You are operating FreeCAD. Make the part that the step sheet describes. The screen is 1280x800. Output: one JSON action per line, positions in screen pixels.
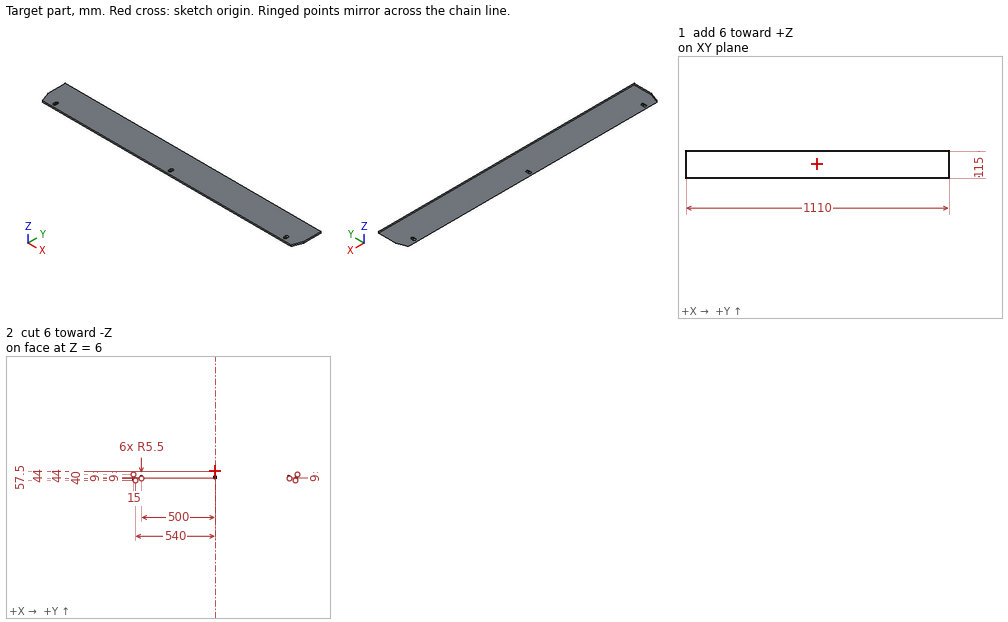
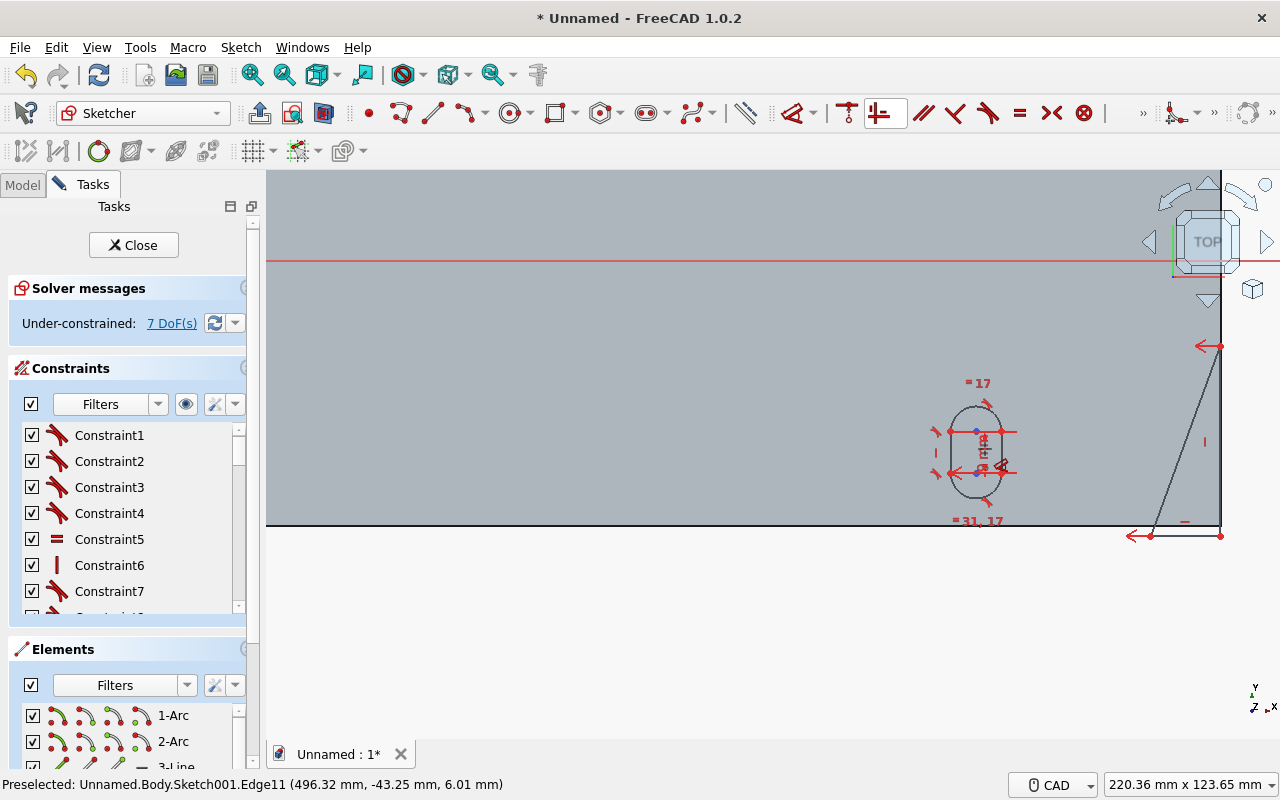
{"action": "scroll", "coordinate": [958, 462], "scroll_direction": "down", "scroll_amount": 11}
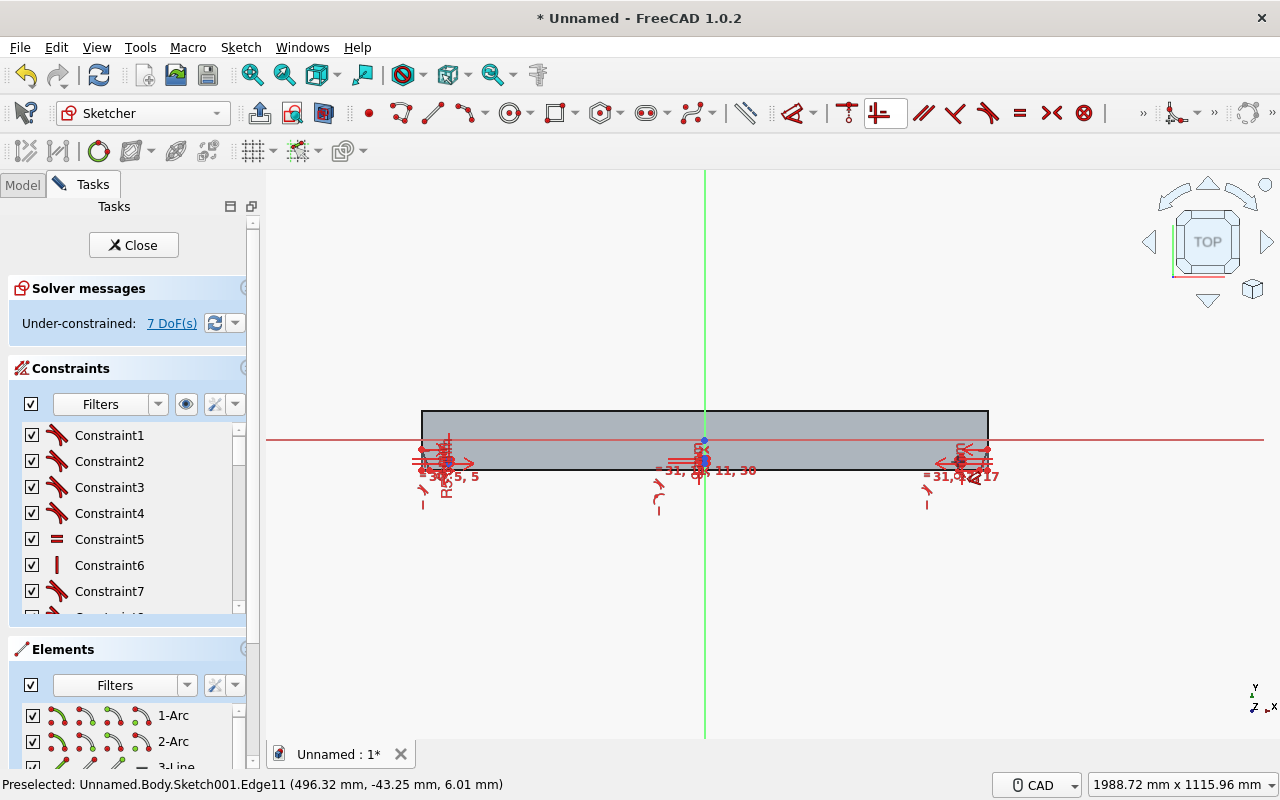
{"action": "scroll", "coordinate": [422, 456], "scroll_direction": "up", "scroll_amount": 10}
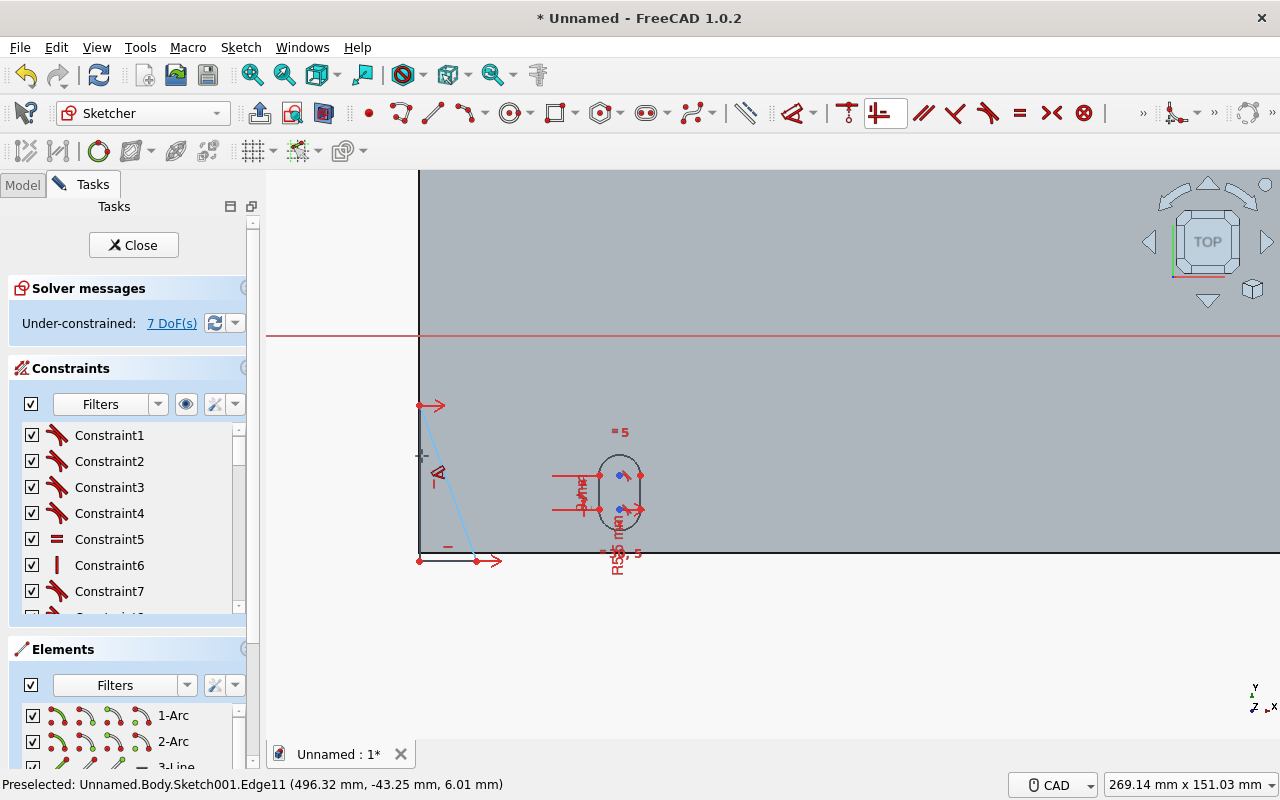
{"action": "left_click", "coordinate": [420, 452]}
{"action": "left_click", "coordinate": [386, 483]}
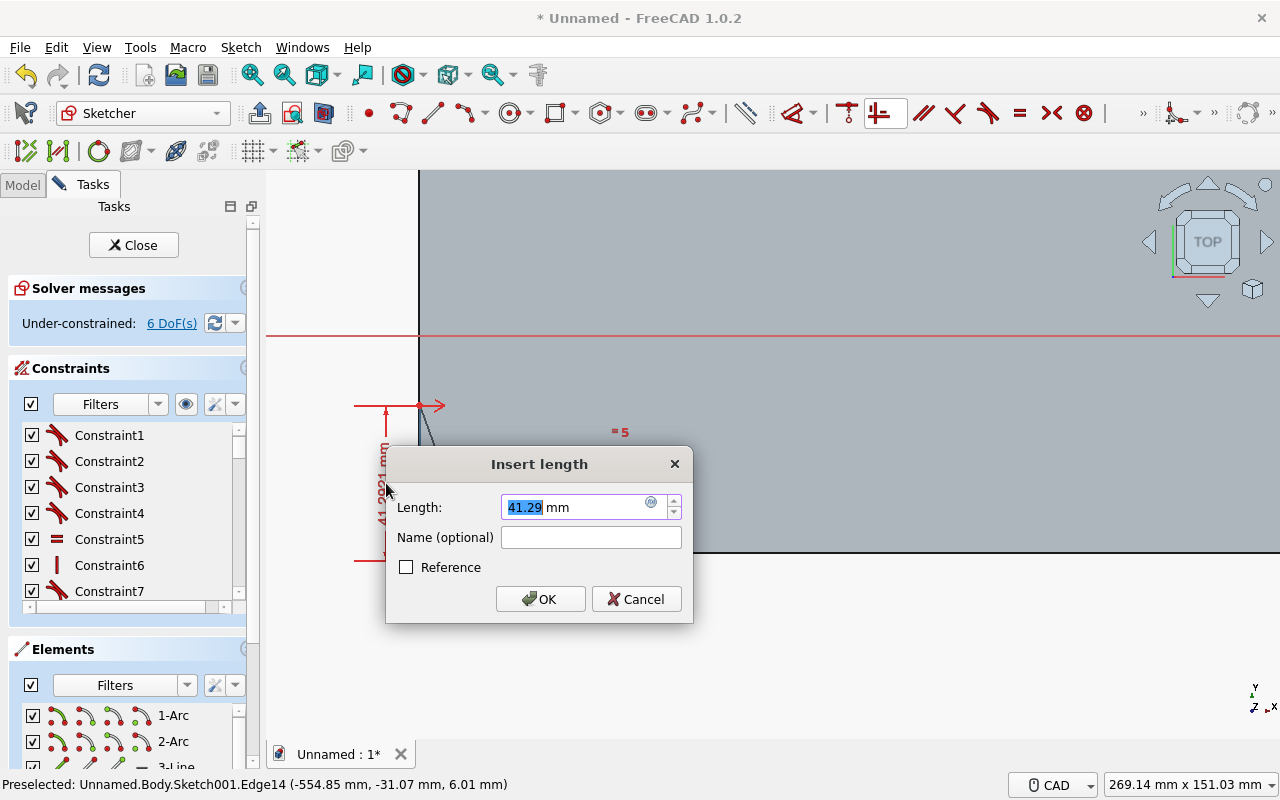
{"action": "type", "text": "40"}
{"action": "key", "text": "Return"}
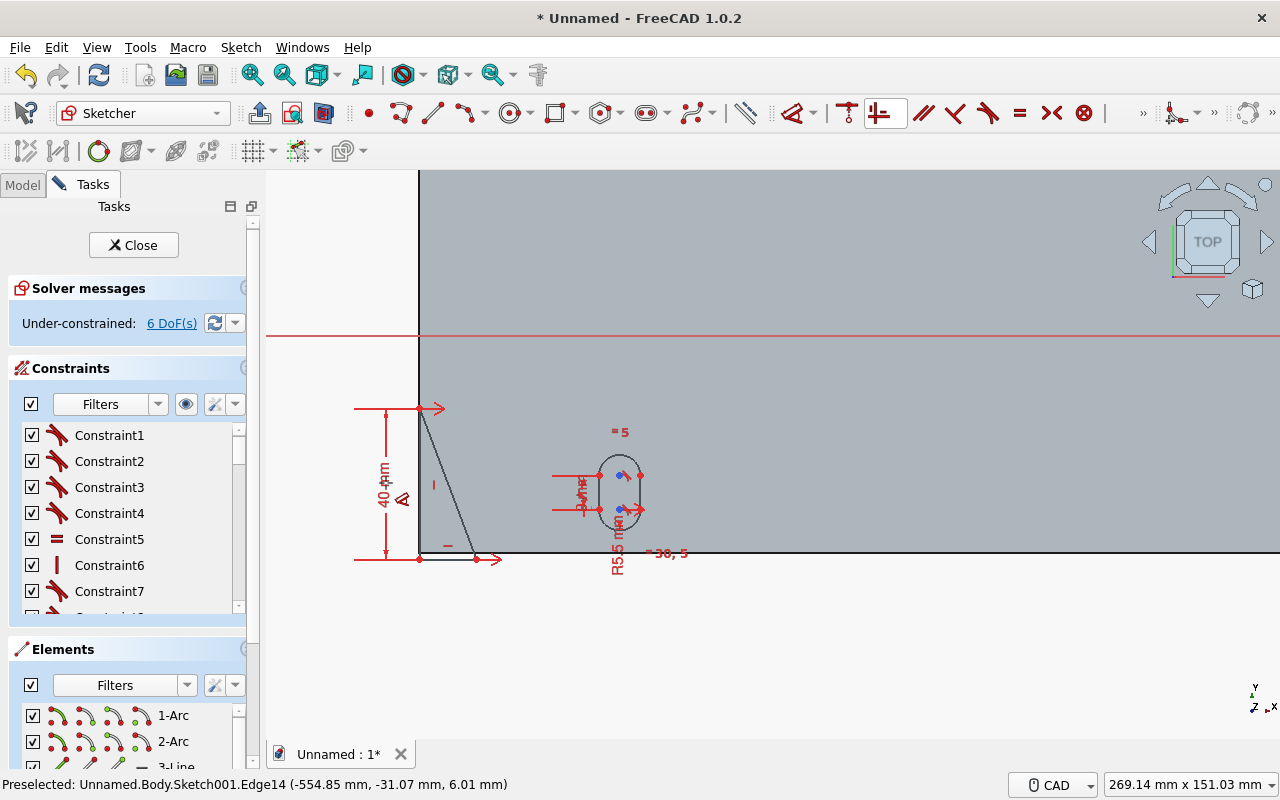
{"action": "left_click", "coordinate": [437, 560]}
{"action": "left_click", "coordinate": [448, 594]}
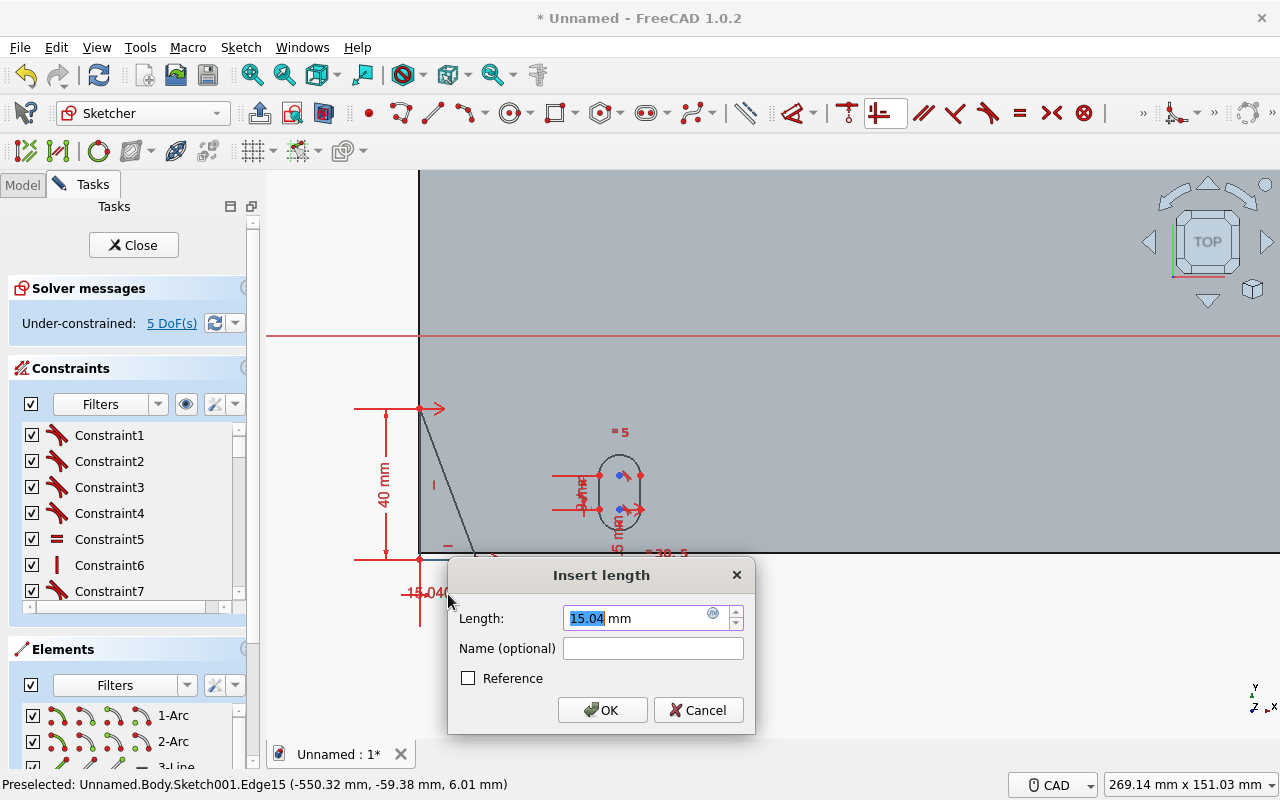
{"action": "type", "text": "15"}
{"action": "key", "text": "Return"}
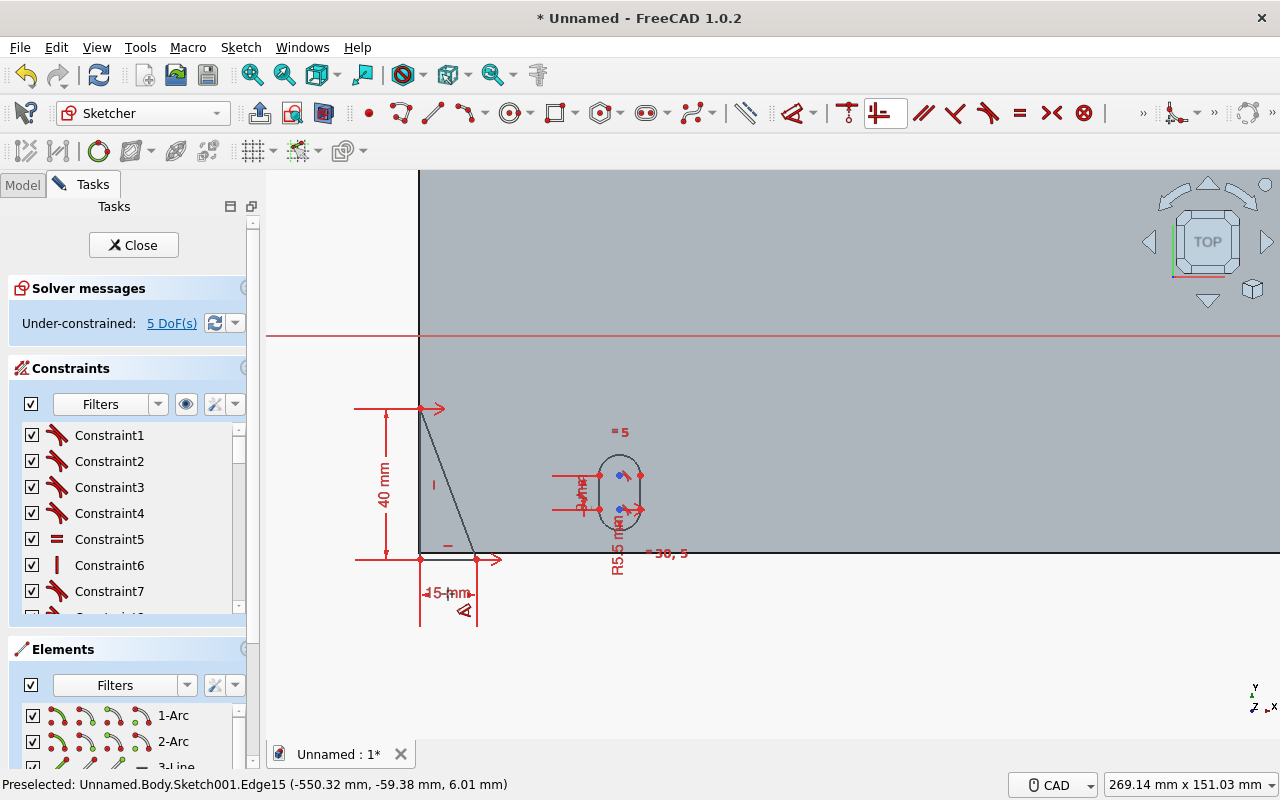
{"action": "left_click", "coordinate": [599, 510]}
{"action": "left_click", "coordinate": [565, 423]}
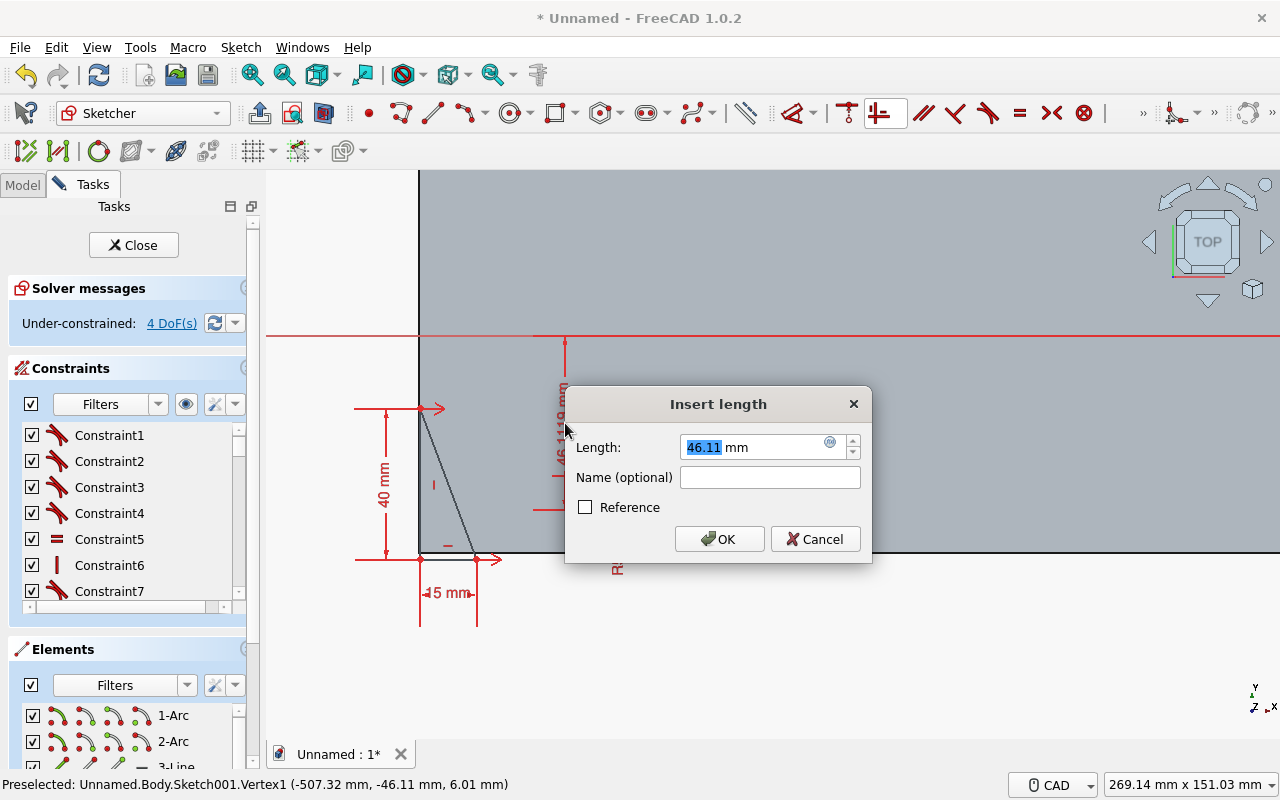
{"action": "type", "text": "44"}
{"action": "key", "text": "Return"}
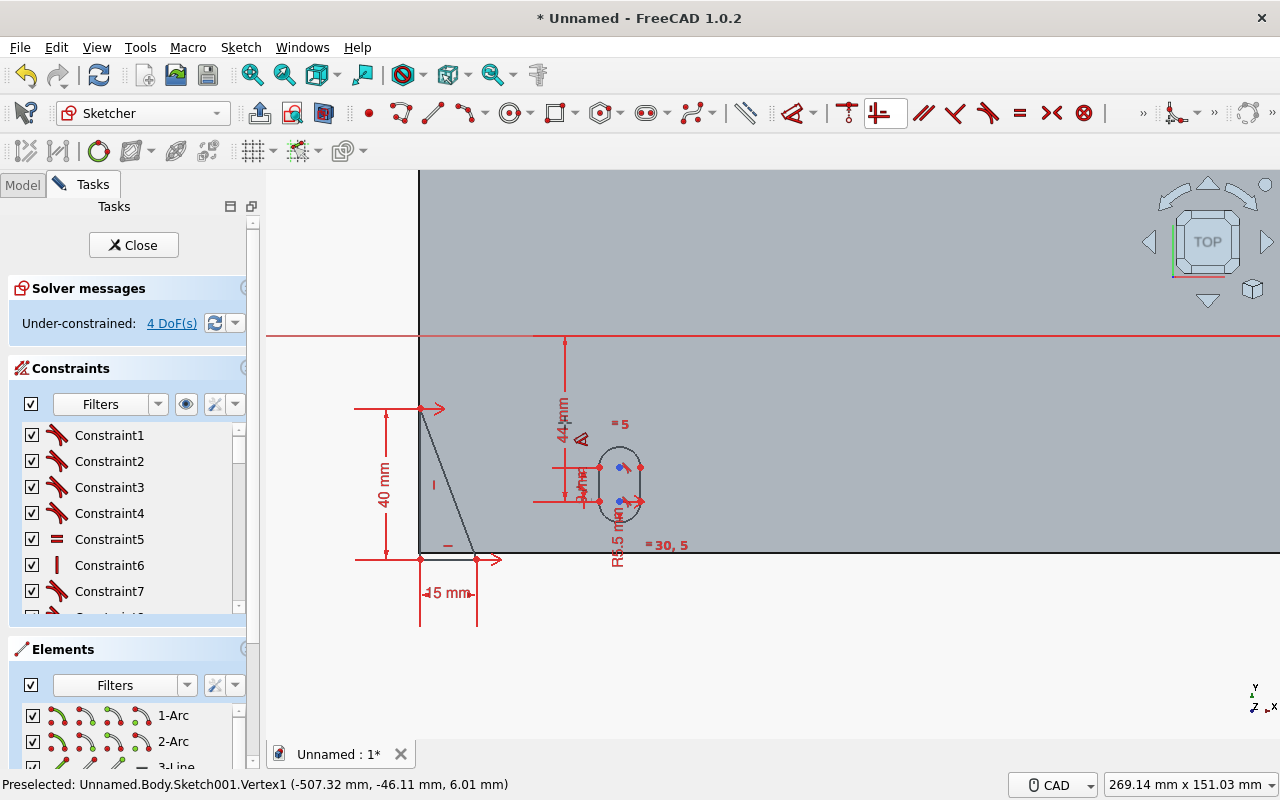
{"action": "scroll", "coordinate": [422, 456], "scroll_direction": "down", "scroll_amount": 10}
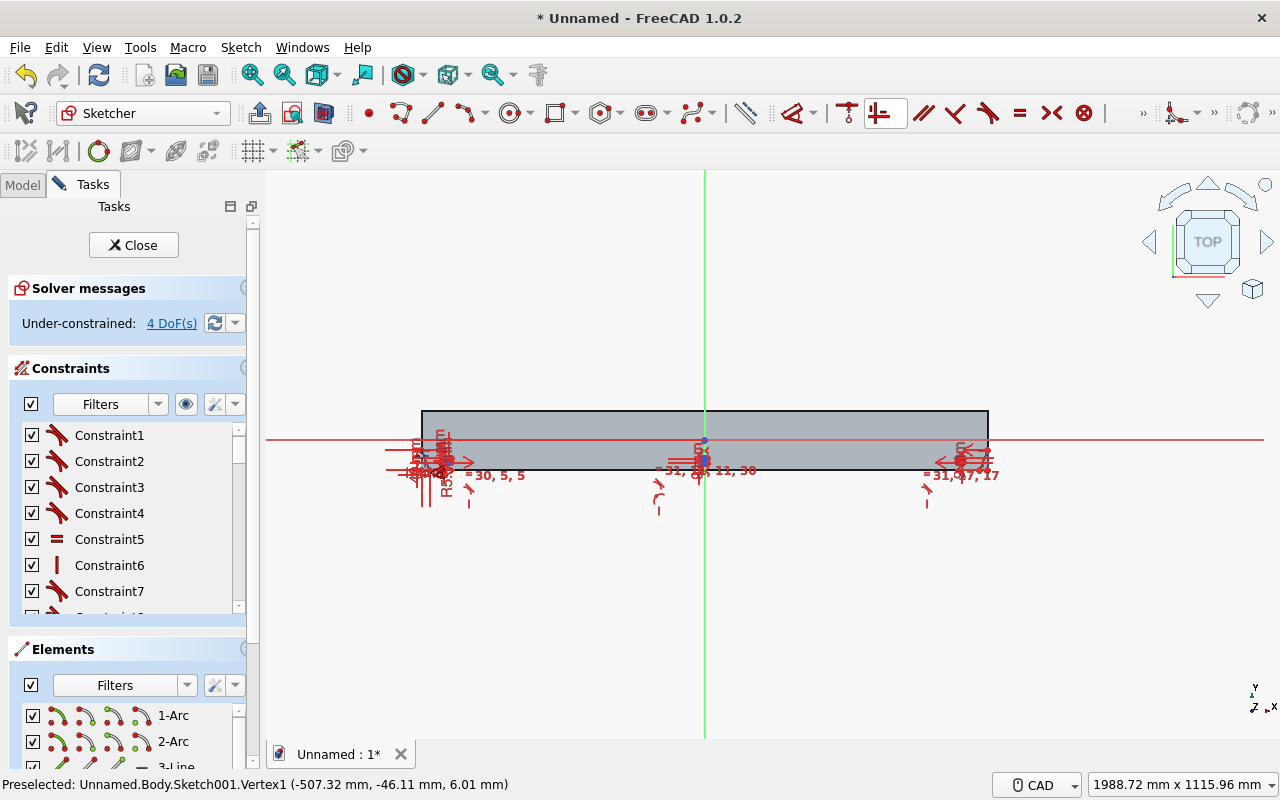
{"action": "scroll", "coordinate": [702, 463], "scroll_direction": "up", "scroll_amount": 8}